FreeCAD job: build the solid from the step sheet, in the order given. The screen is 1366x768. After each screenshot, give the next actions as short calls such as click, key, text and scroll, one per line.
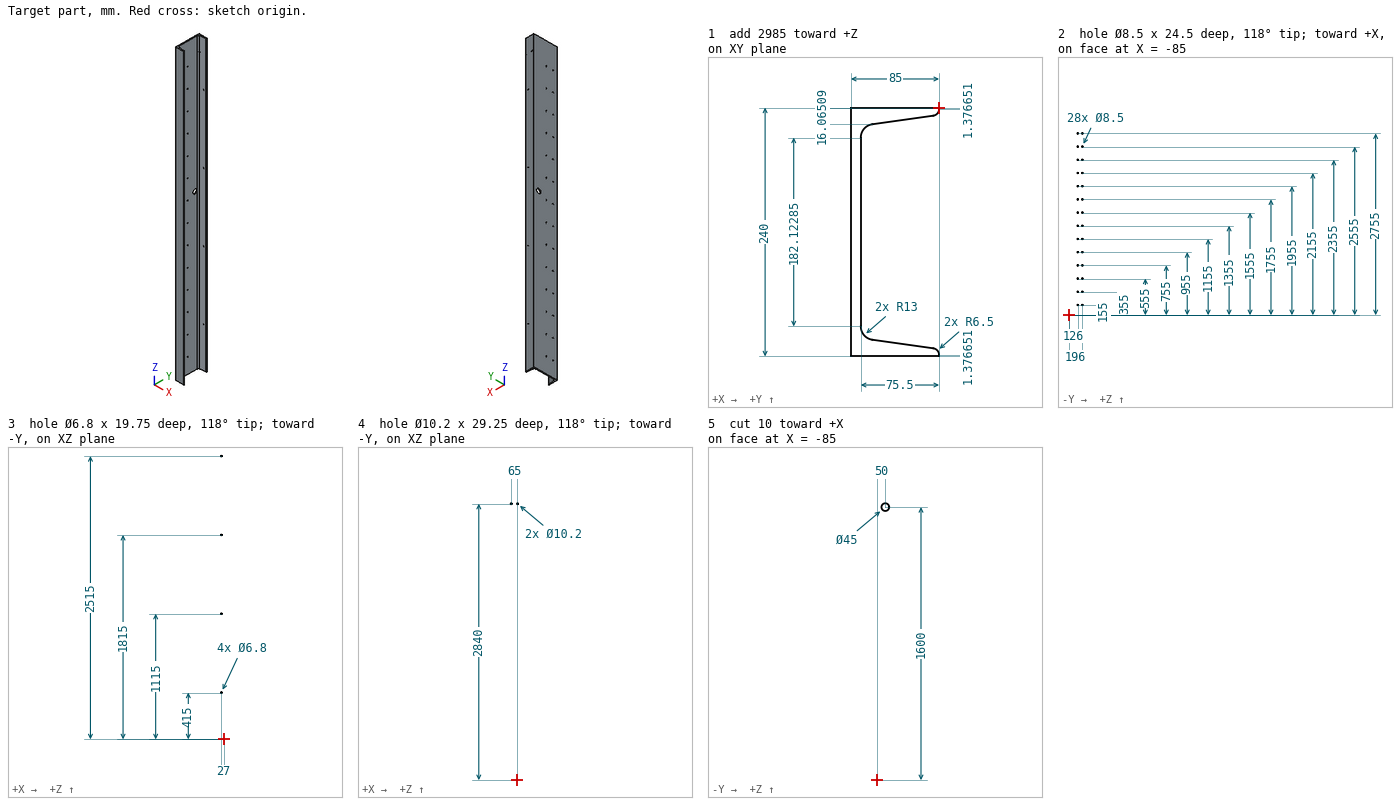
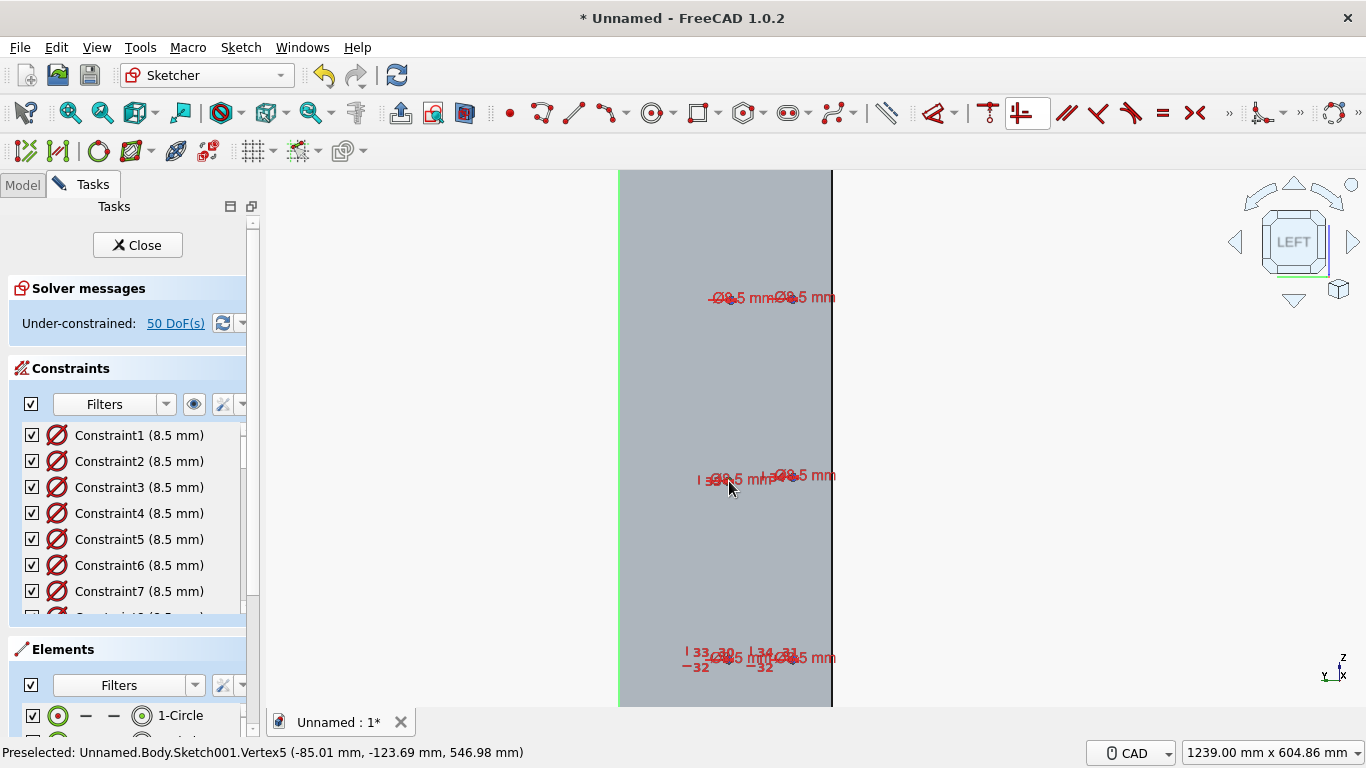
scroll(754, 547, down, 10)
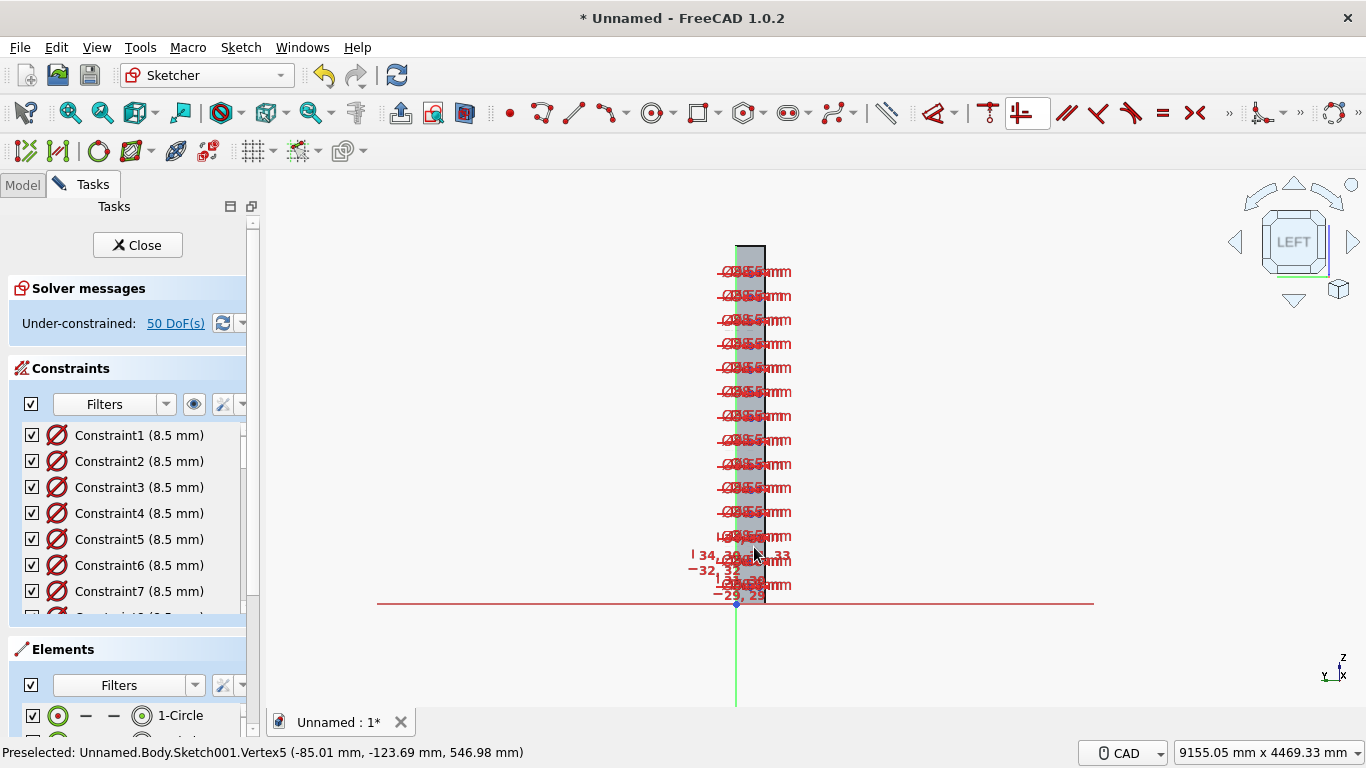
scroll(760, 538, up, 2)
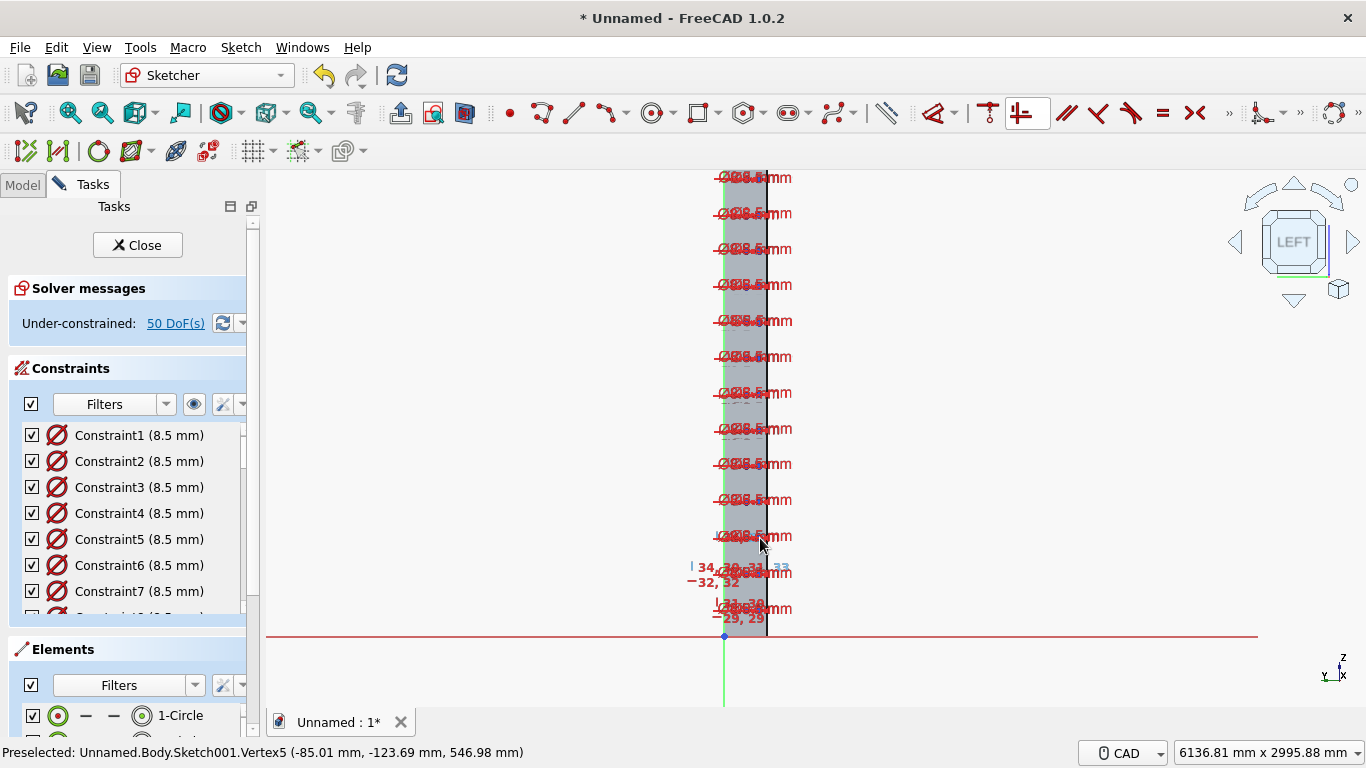
scroll(759, 538, up, 4)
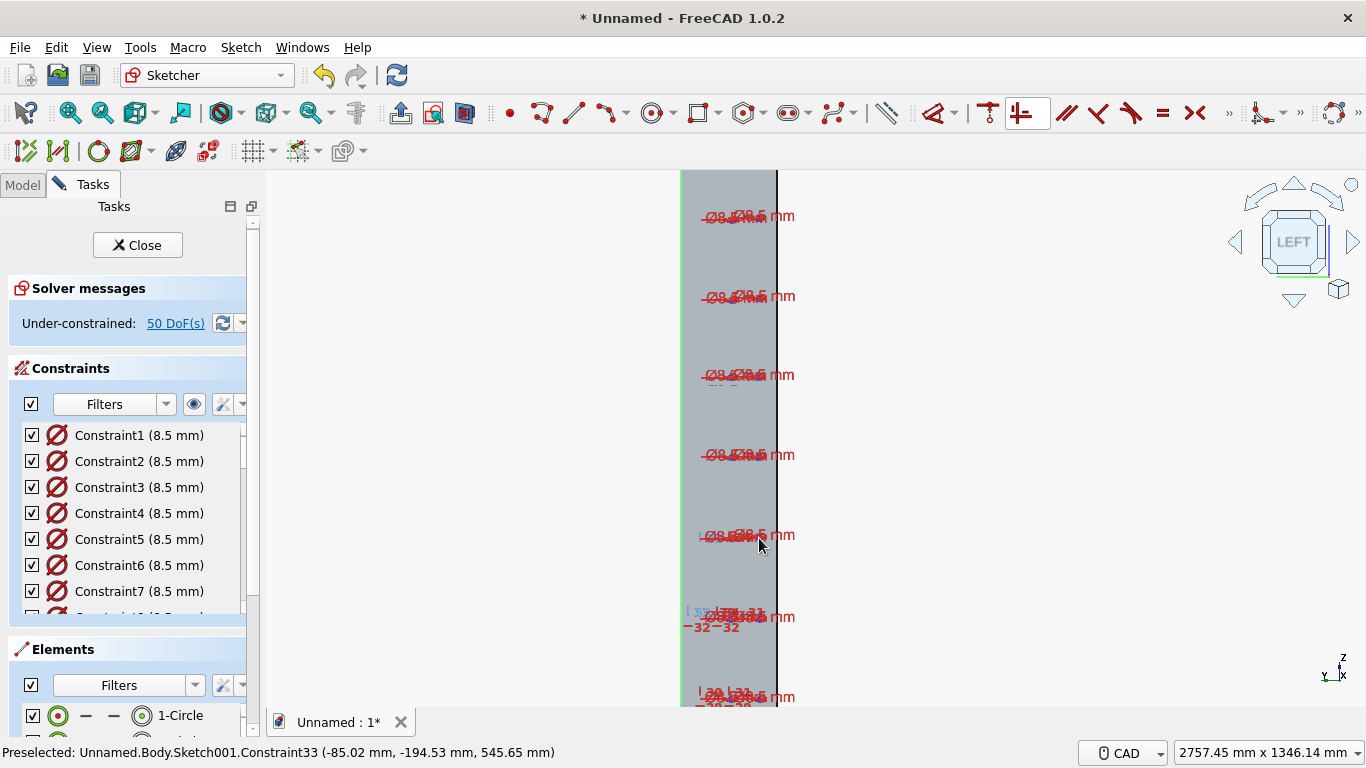
click(759, 537)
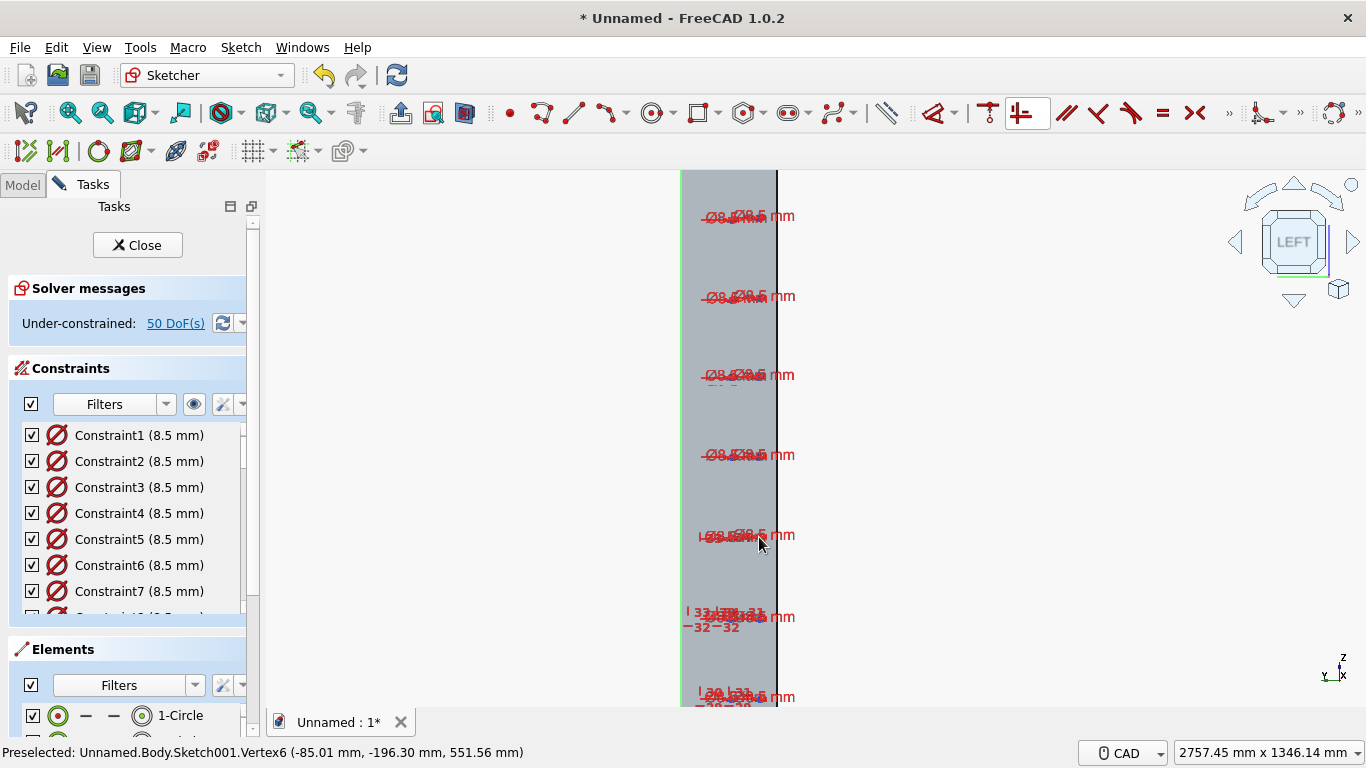
key(h)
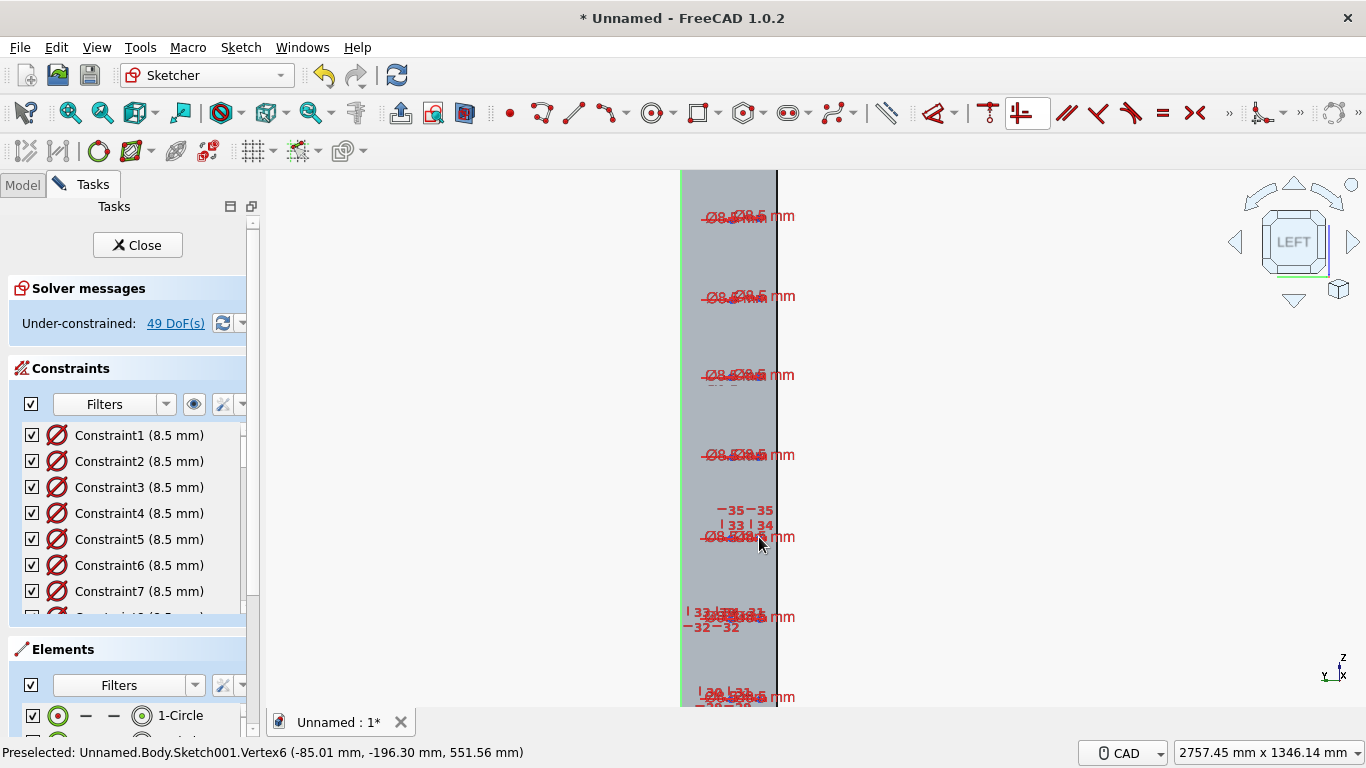
click(730, 539)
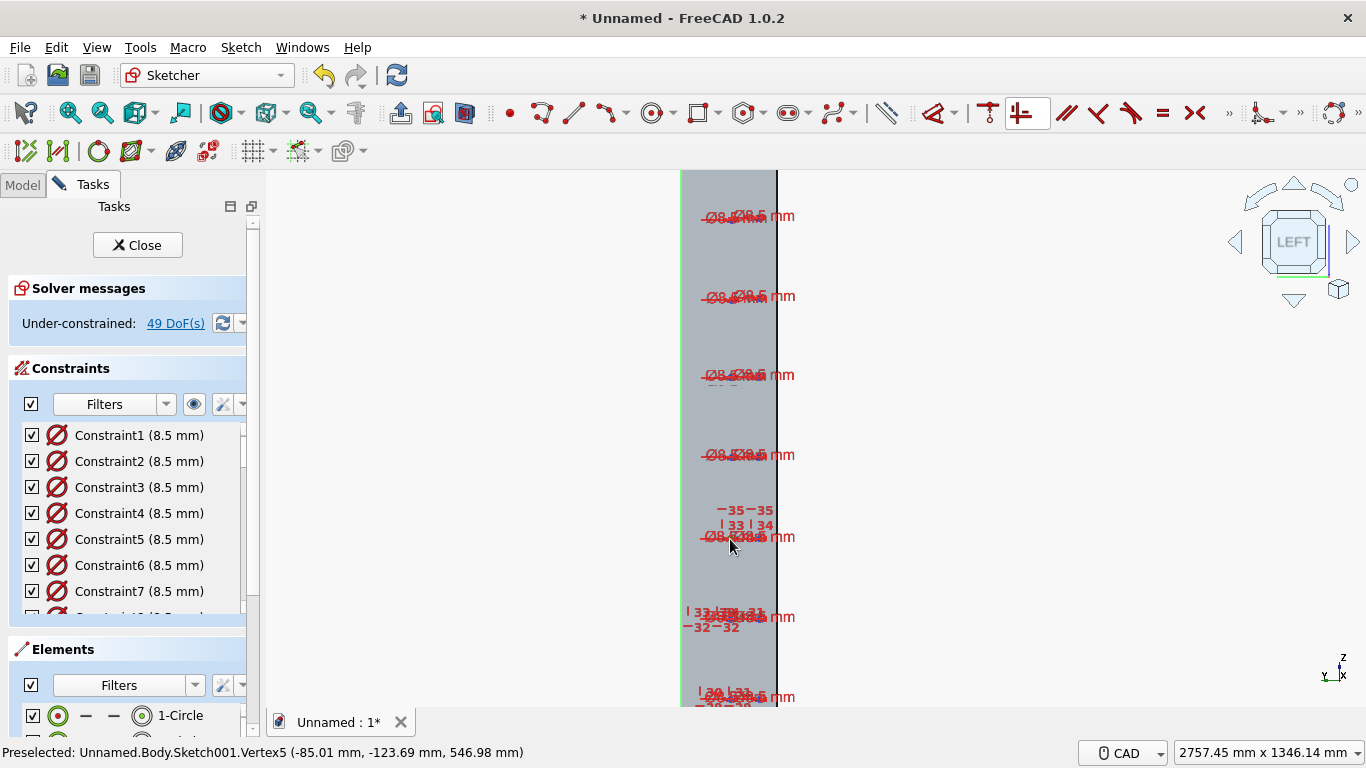
click(731, 457)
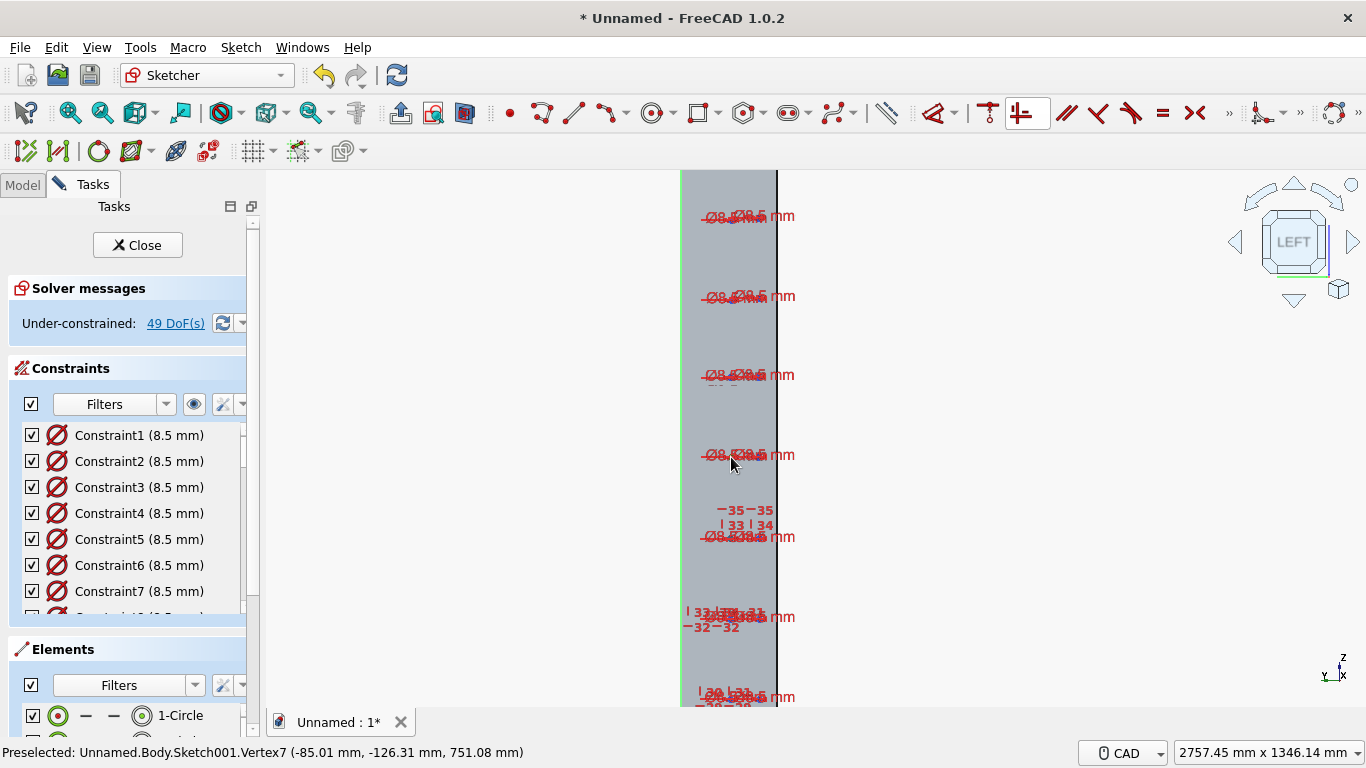
click(1044, 114)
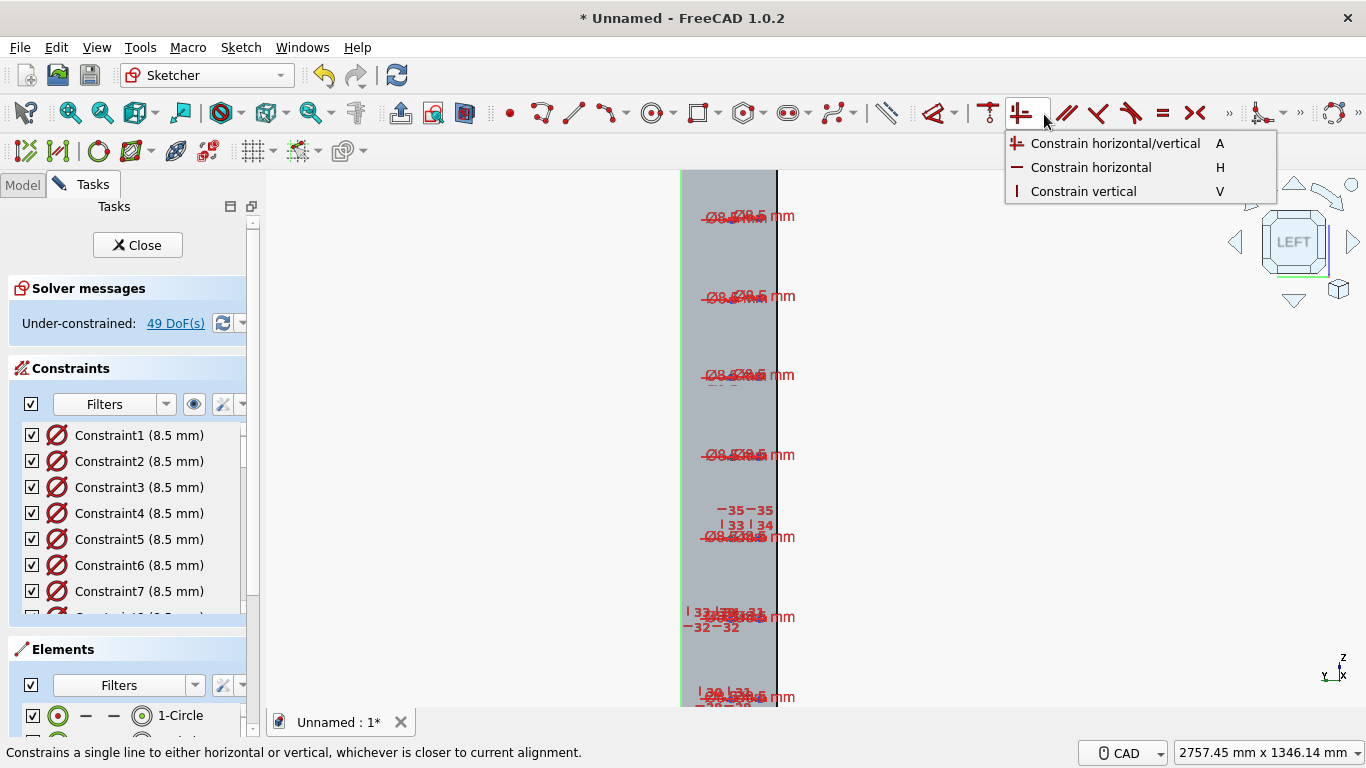
click(1141, 191)